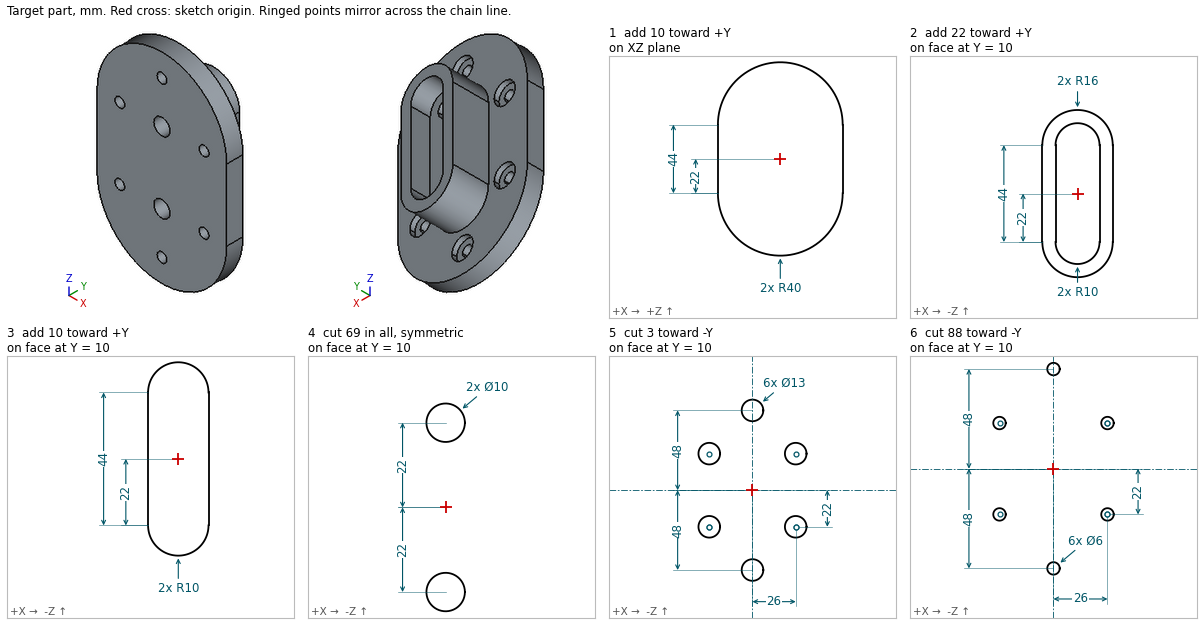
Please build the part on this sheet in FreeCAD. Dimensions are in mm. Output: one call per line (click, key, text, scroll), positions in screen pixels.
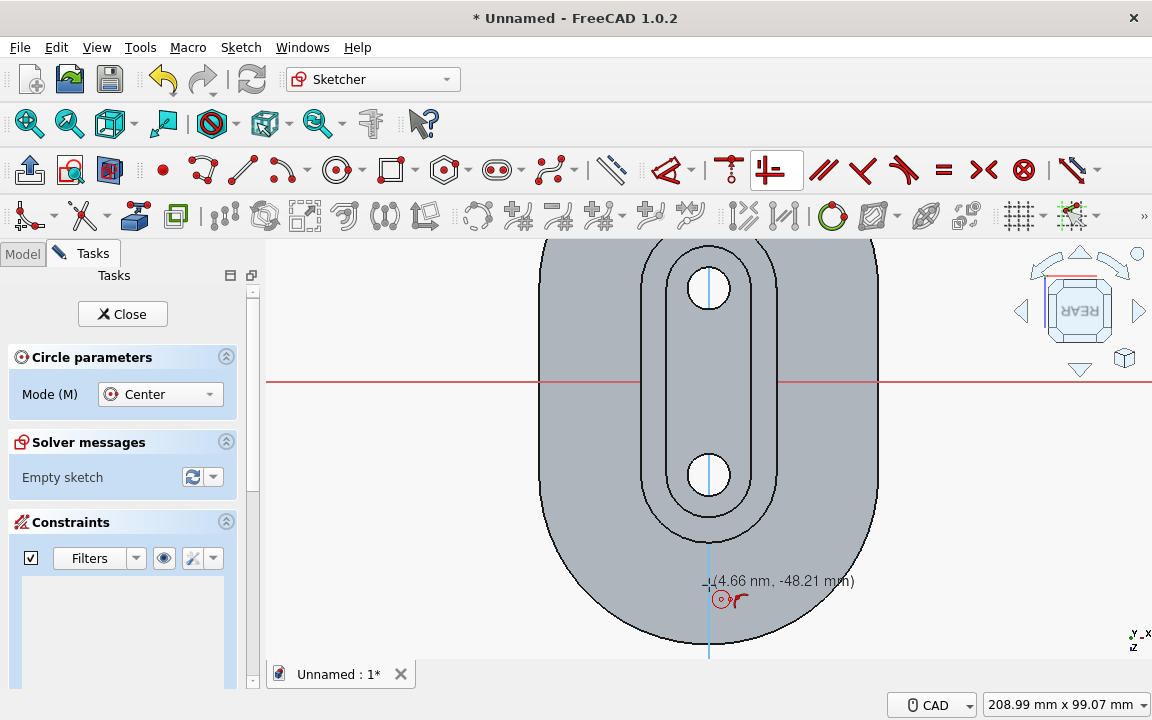
click(709, 585)
move(728, 566)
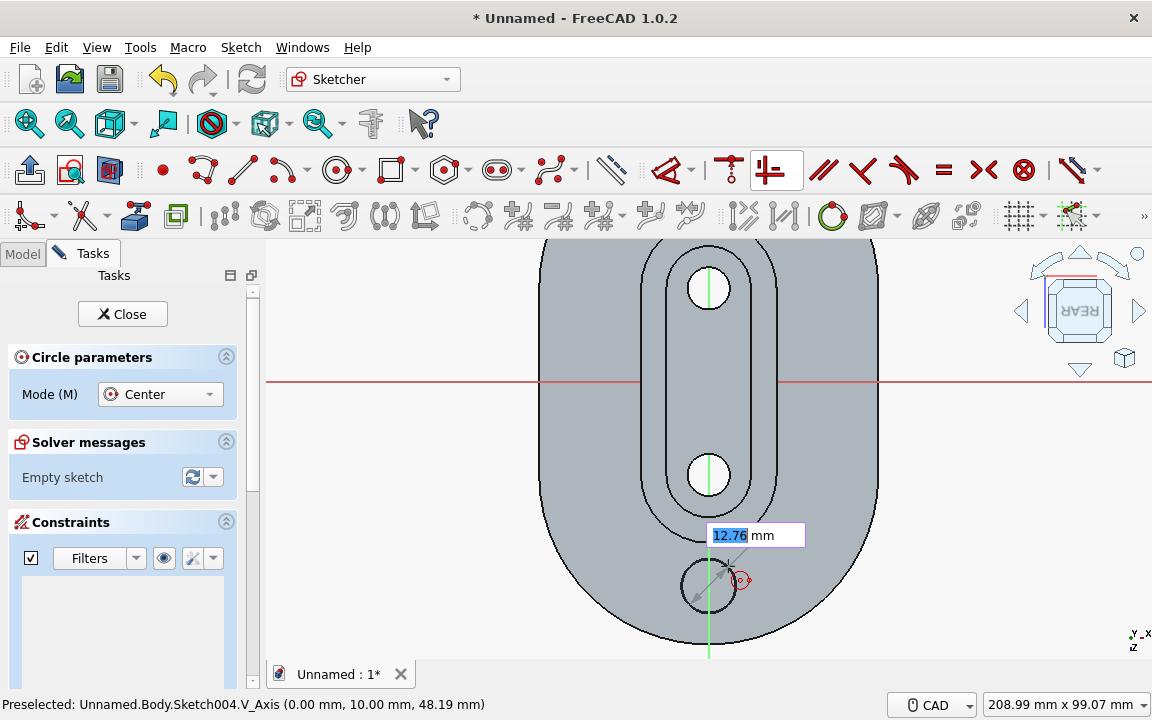
text(13)
key(Return)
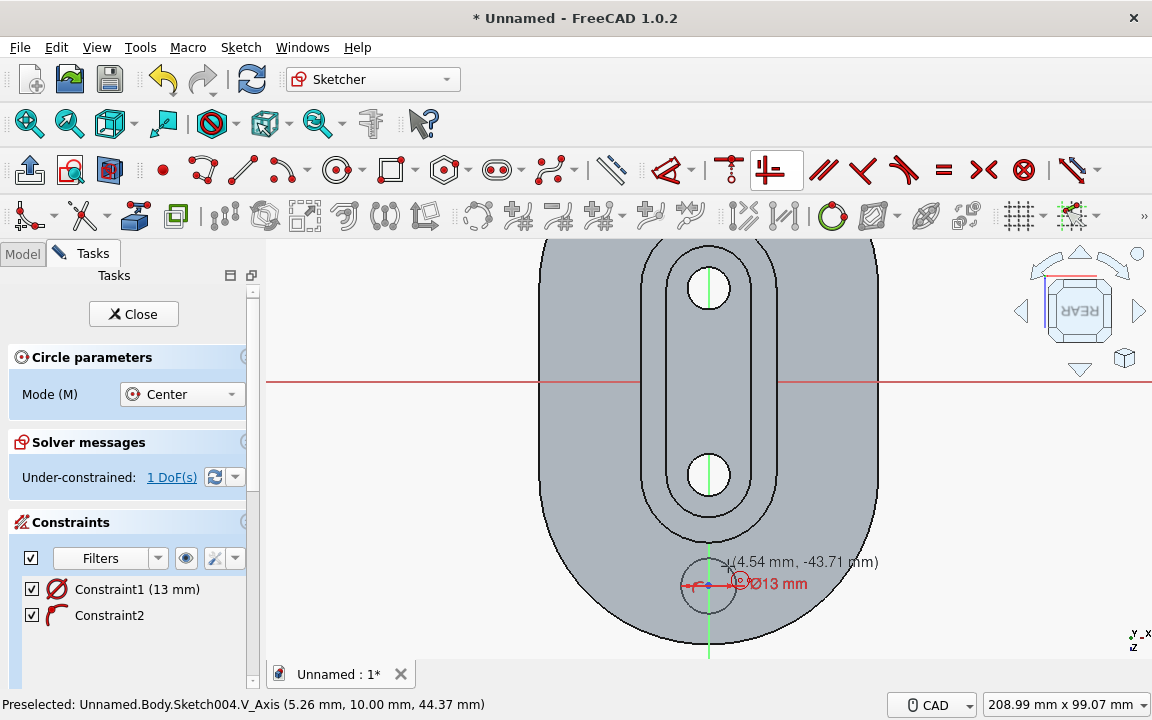
scroll(557, 531, down, 3)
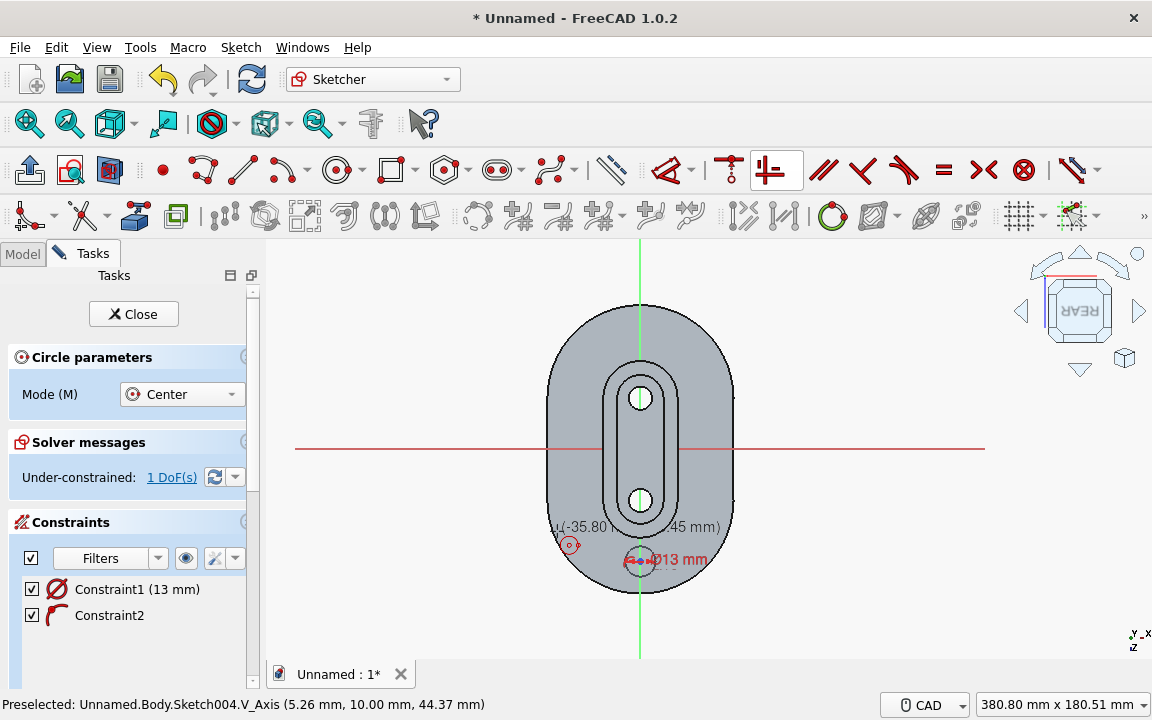
scroll(640, 338, up, 3)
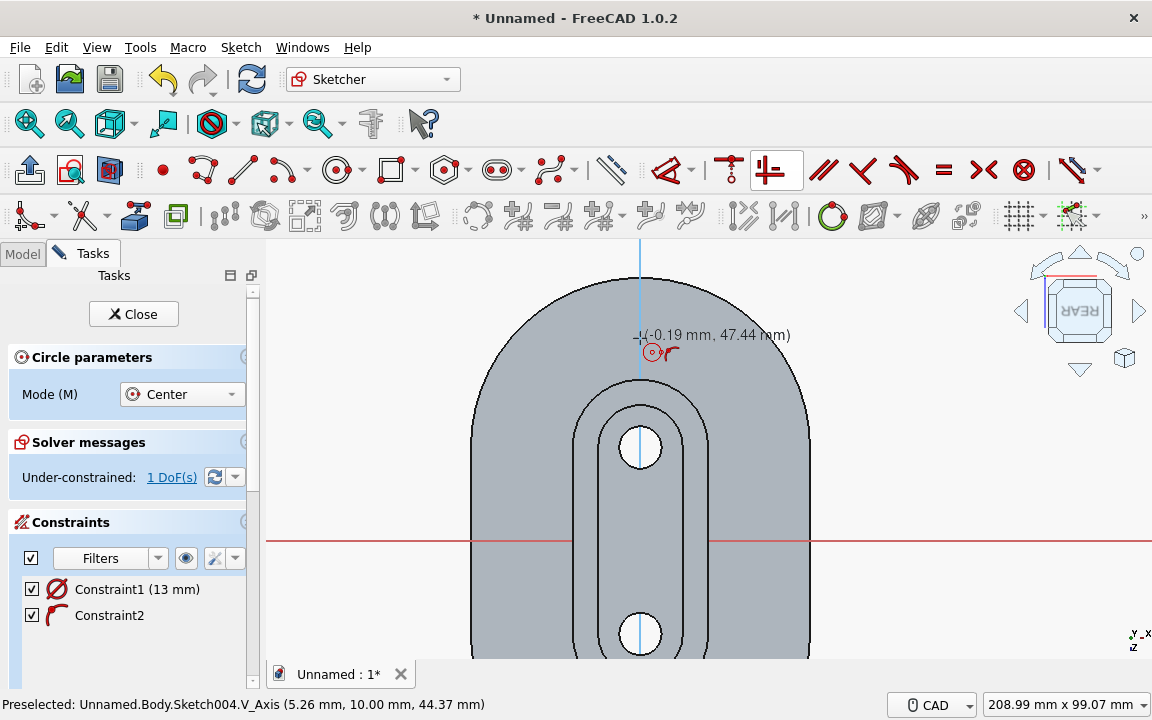
click(640, 337)
move(660, 318)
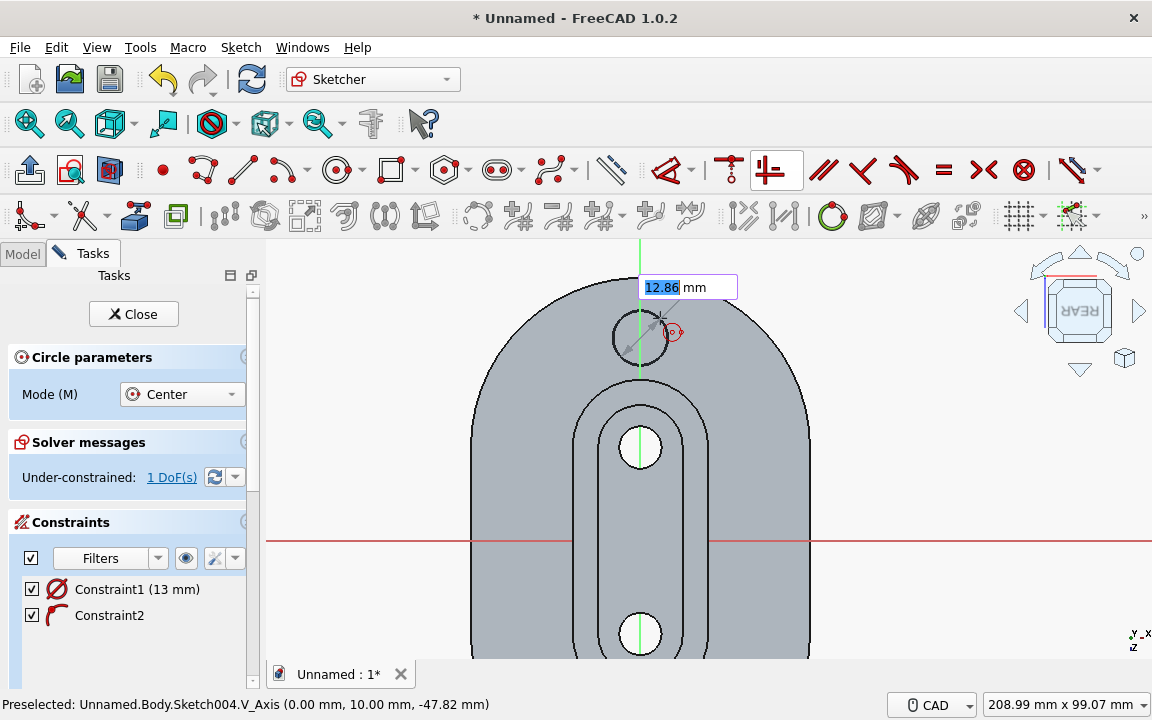
text(13)
key(Return)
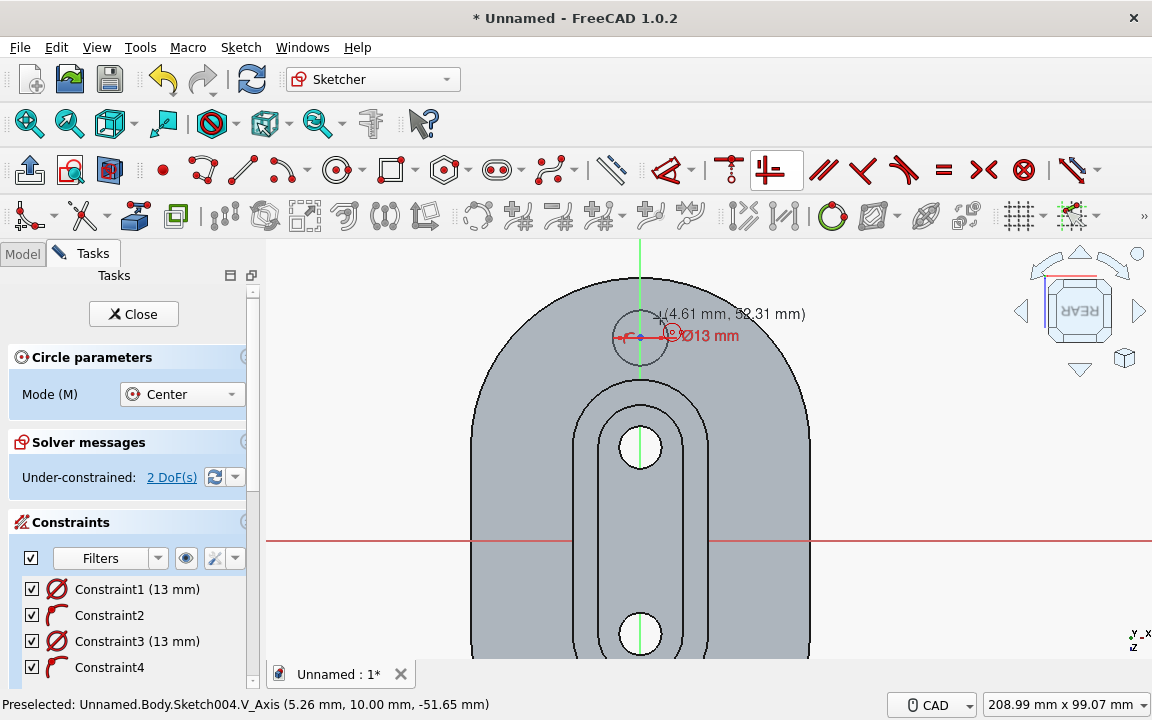
scroll(641, 337, down, 3)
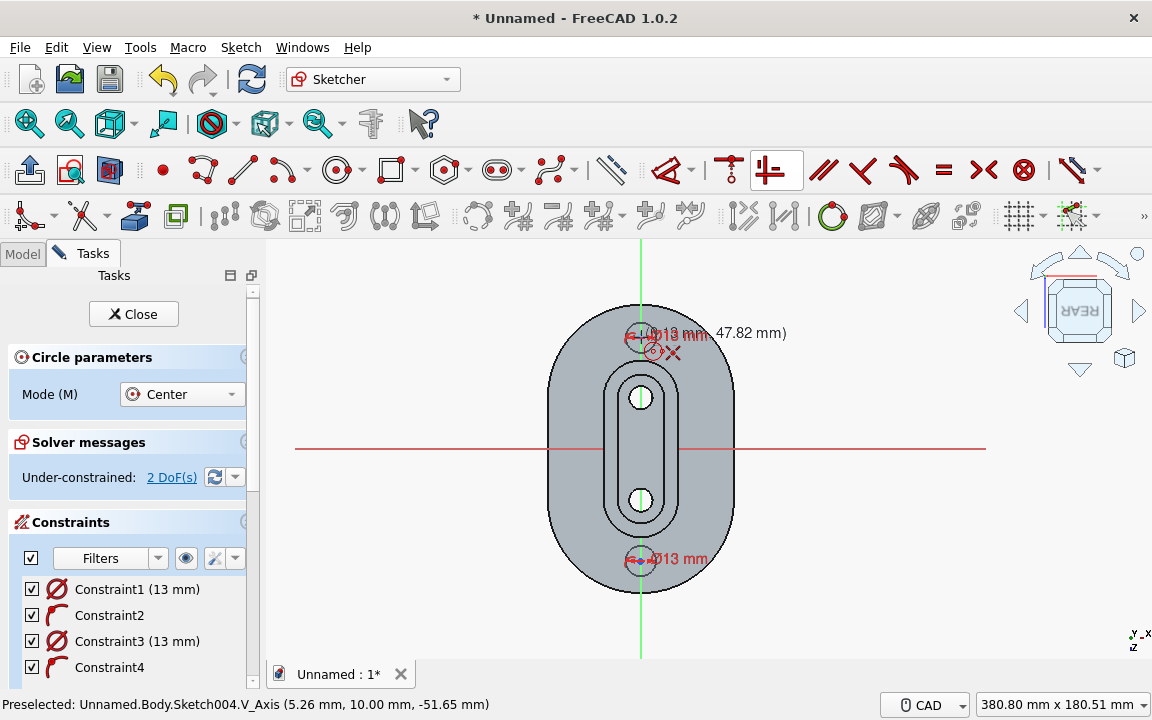
scroll(701, 500, up, 3)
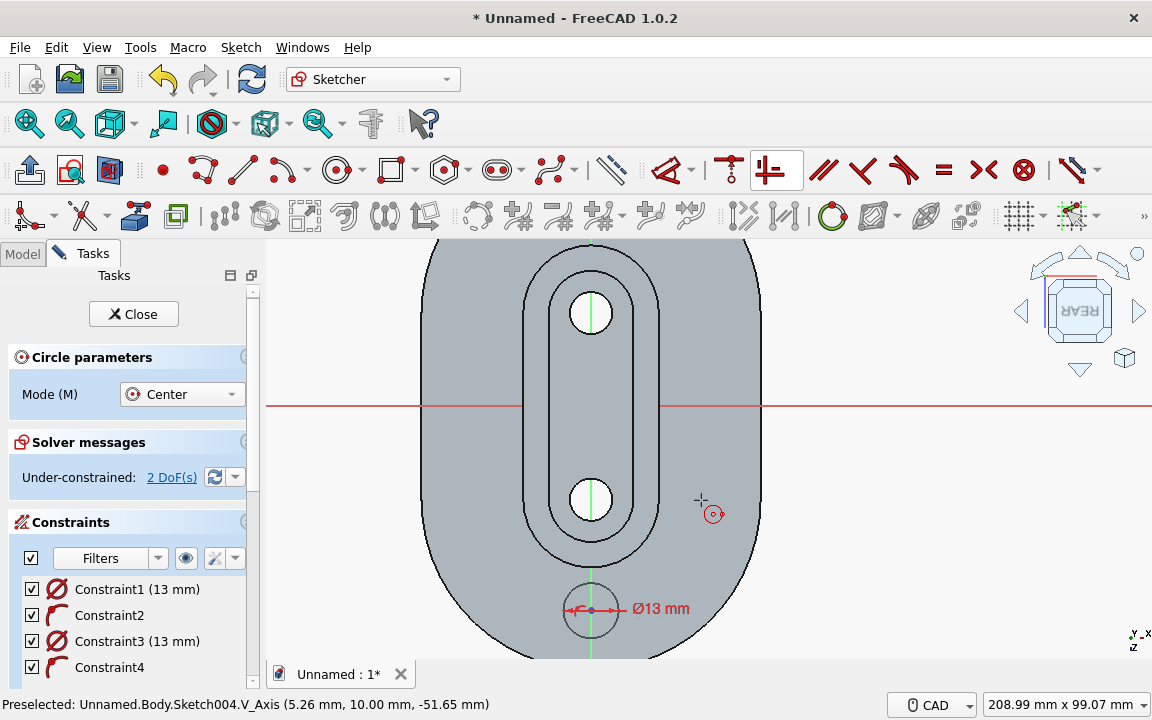
click(701, 500)
move(721, 480)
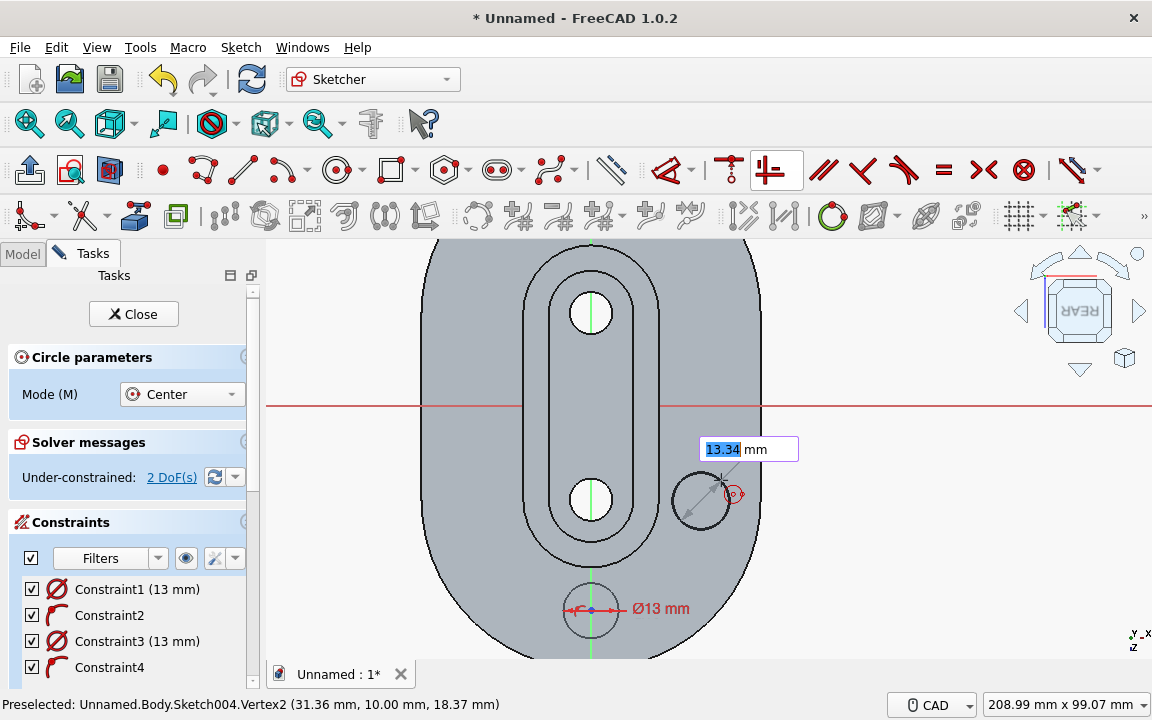
text(13)
key(Return)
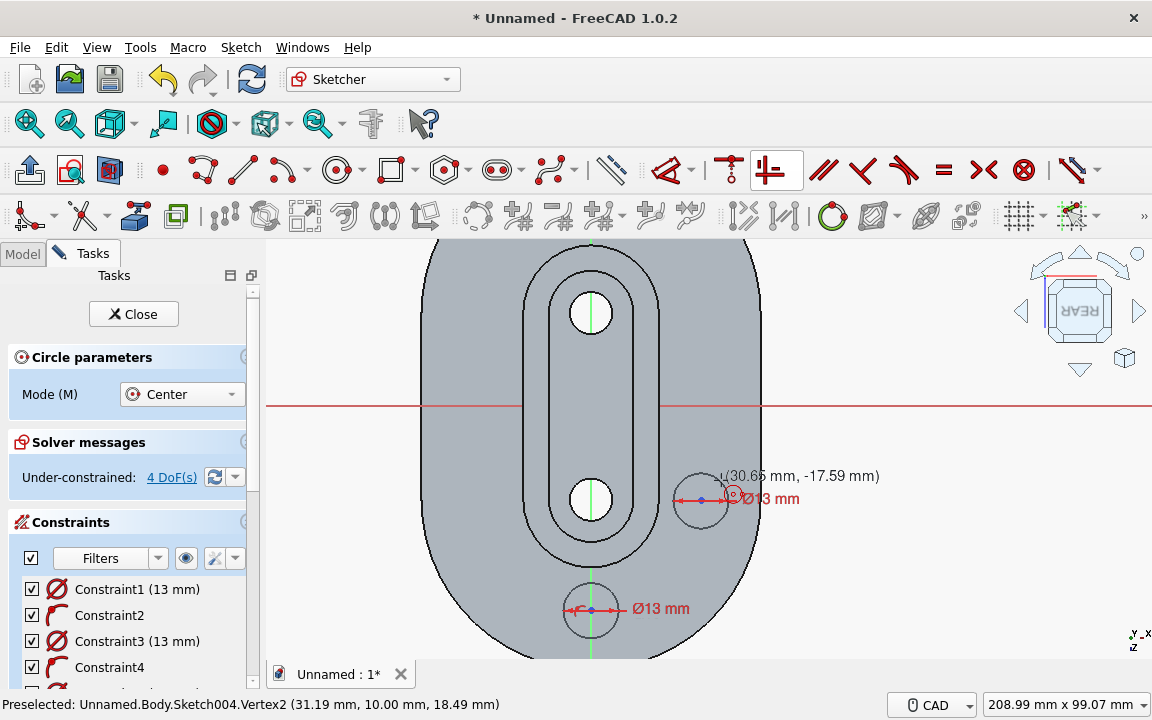
click(481, 500)
move(500, 480)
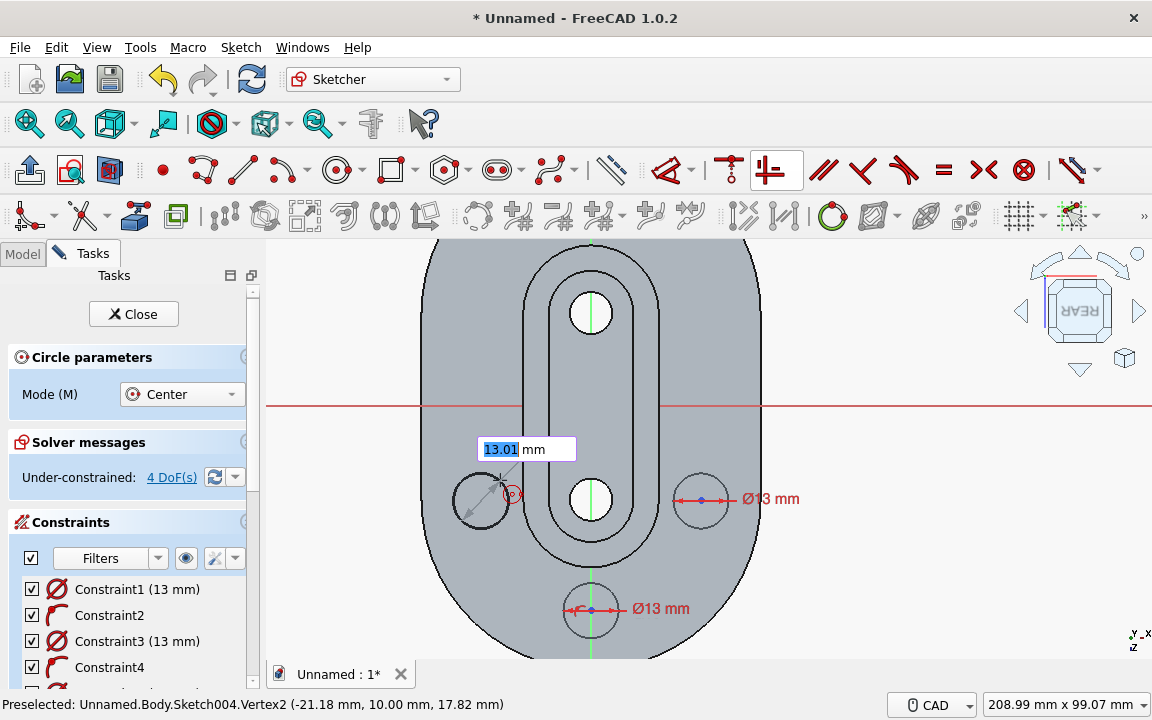
text(13)
key(Return)